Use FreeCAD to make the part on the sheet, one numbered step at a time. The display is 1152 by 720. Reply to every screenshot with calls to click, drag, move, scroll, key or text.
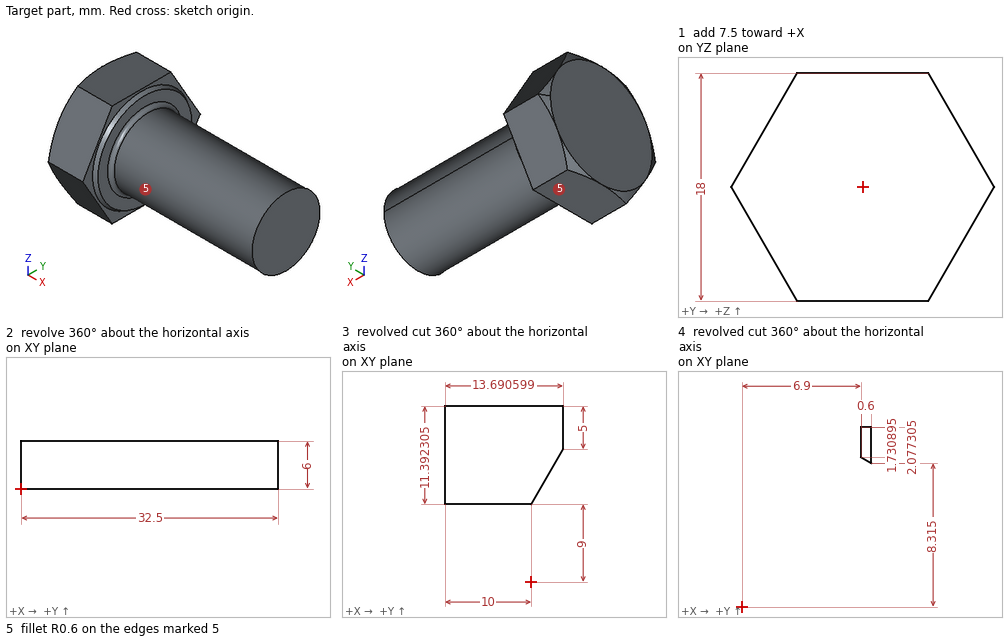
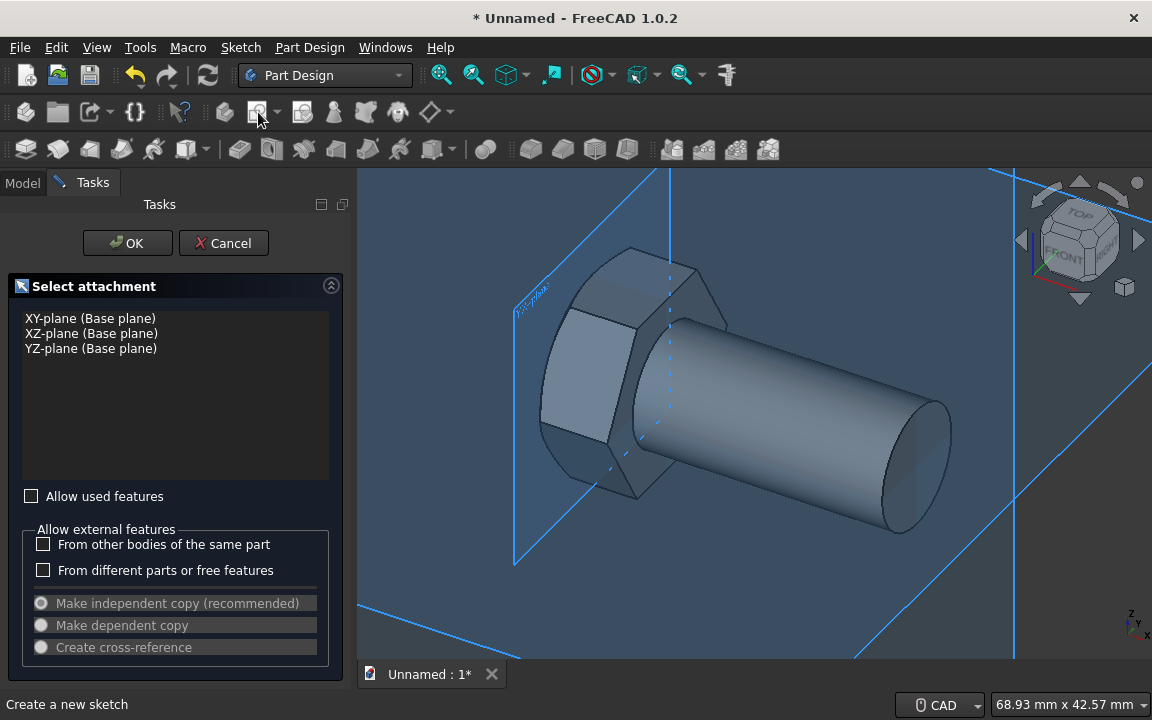
click(82, 318)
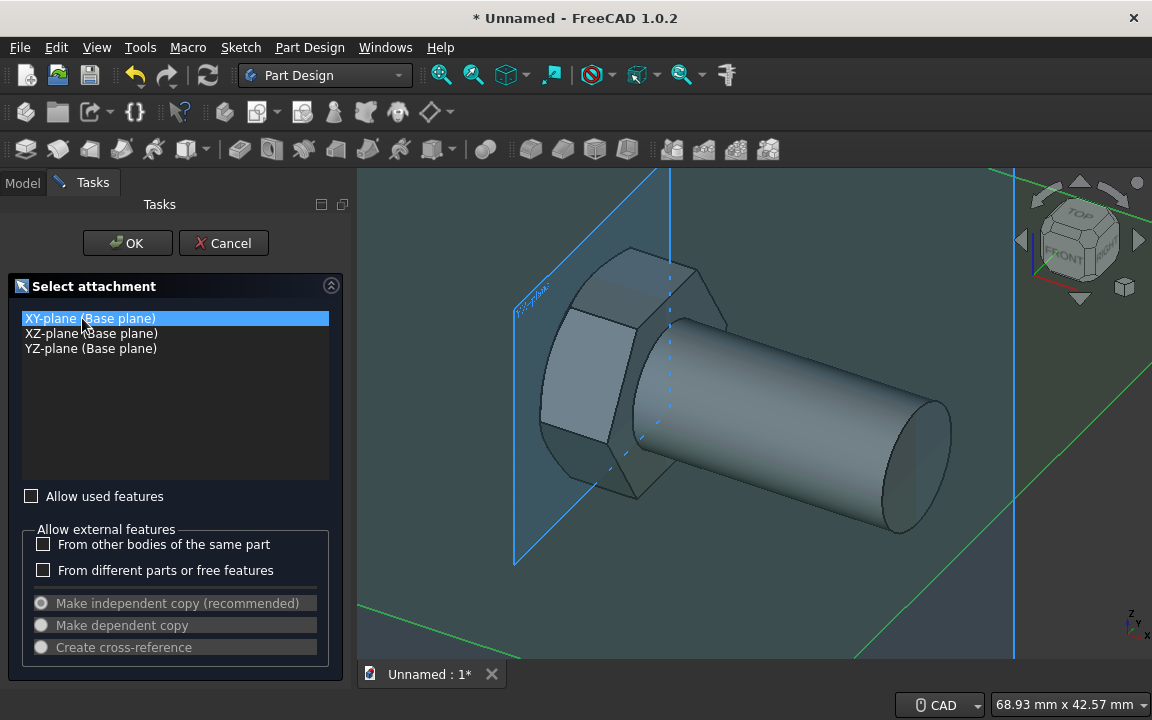
click(128, 243)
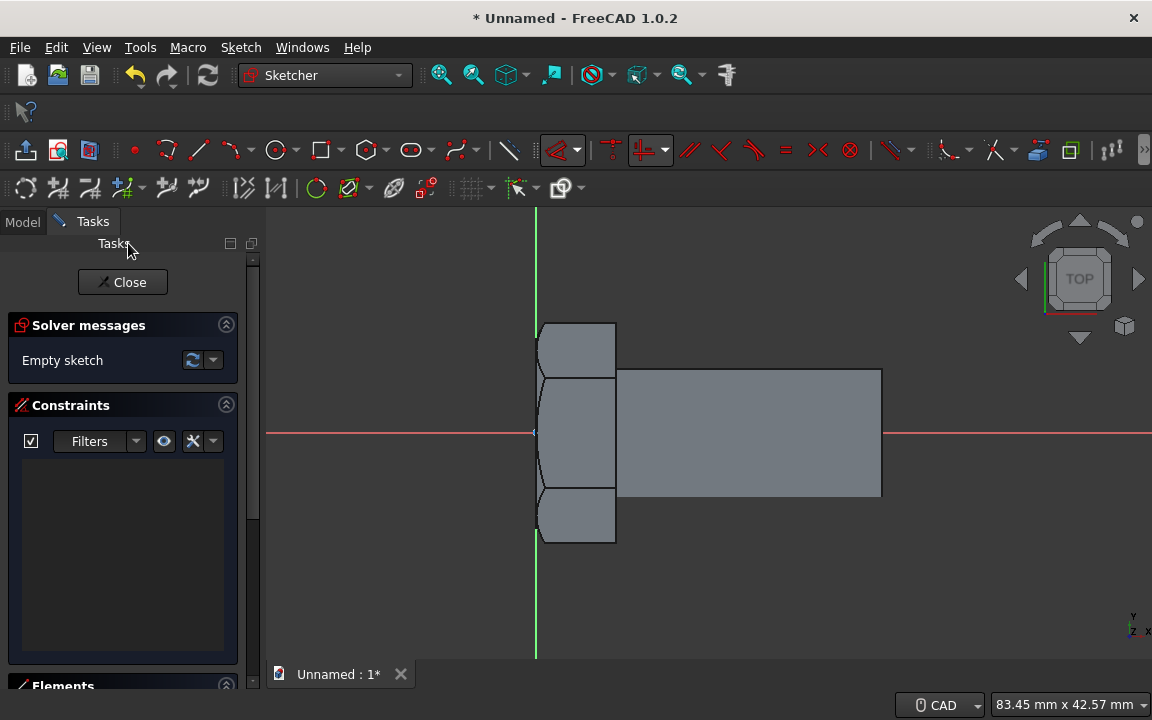
click(90, 150)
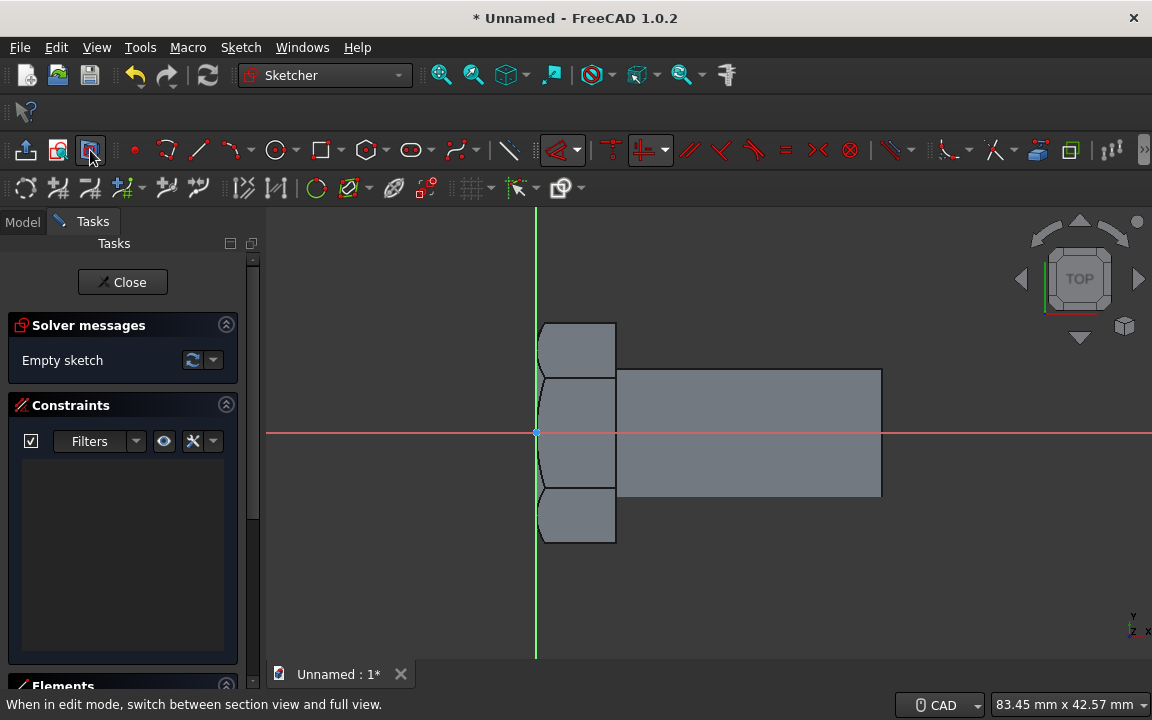
scroll(611, 326, up, 13)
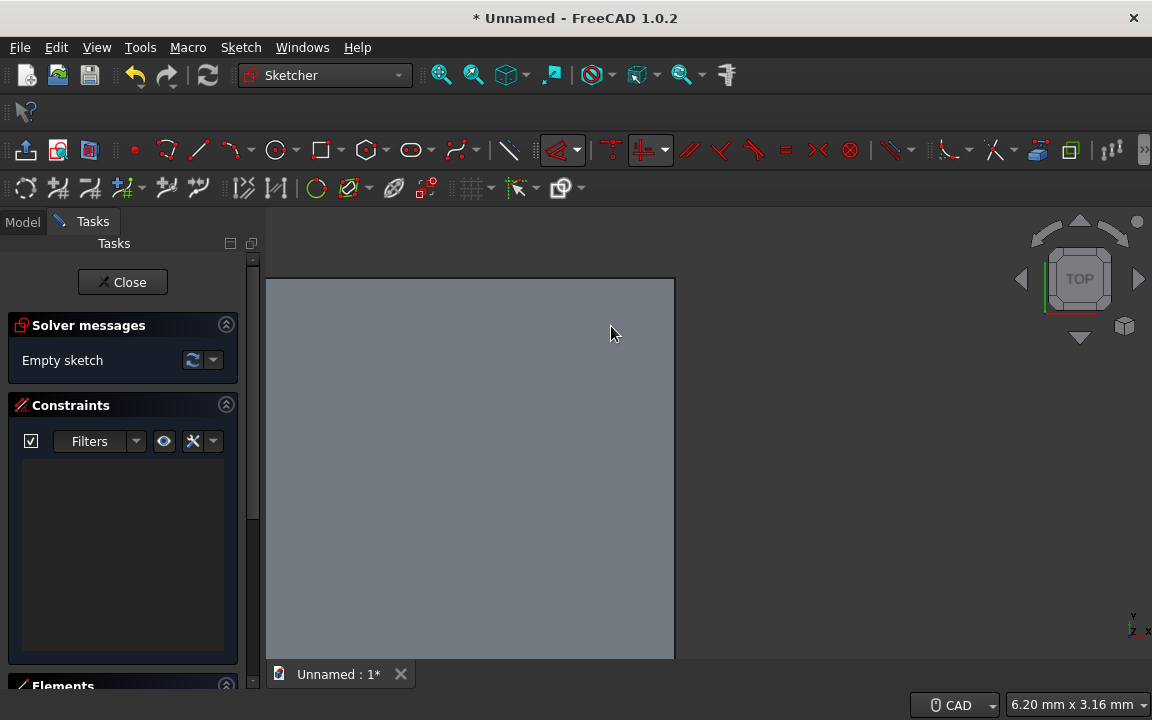
click(168, 150)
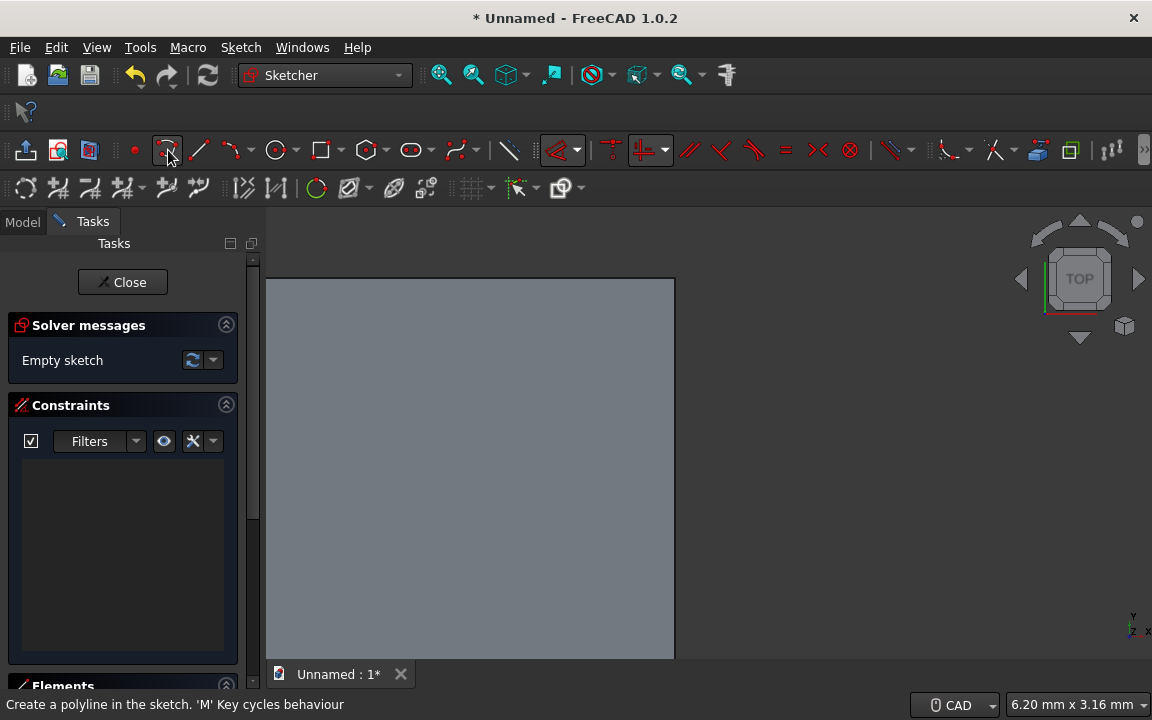
click(589, 525)
click(675, 575)
click(675, 278)
click(589, 278)
click(589, 526)
key(Escape)
key(Escape)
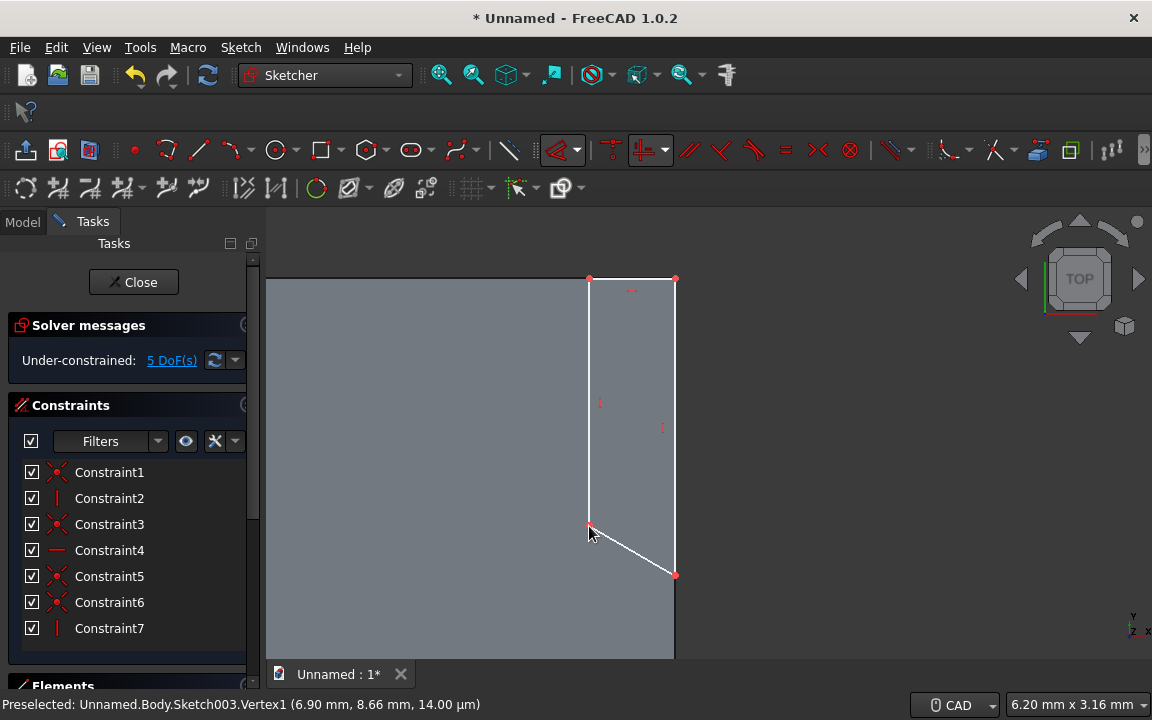
click(649, 279)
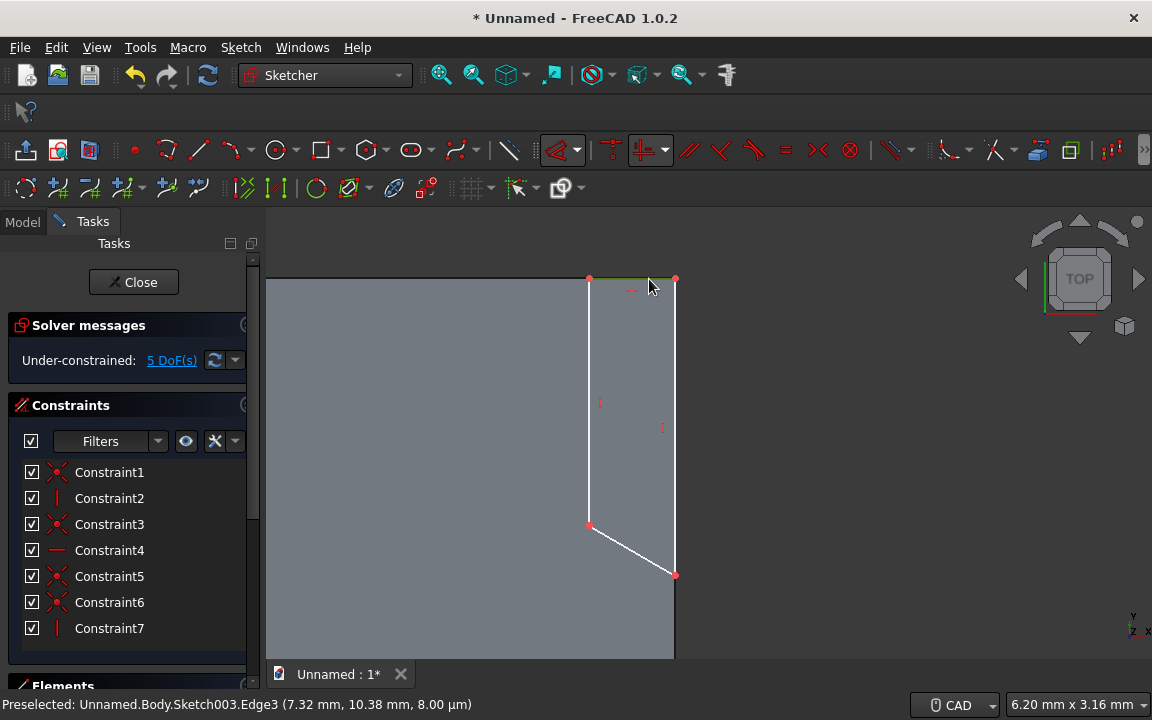
key(l)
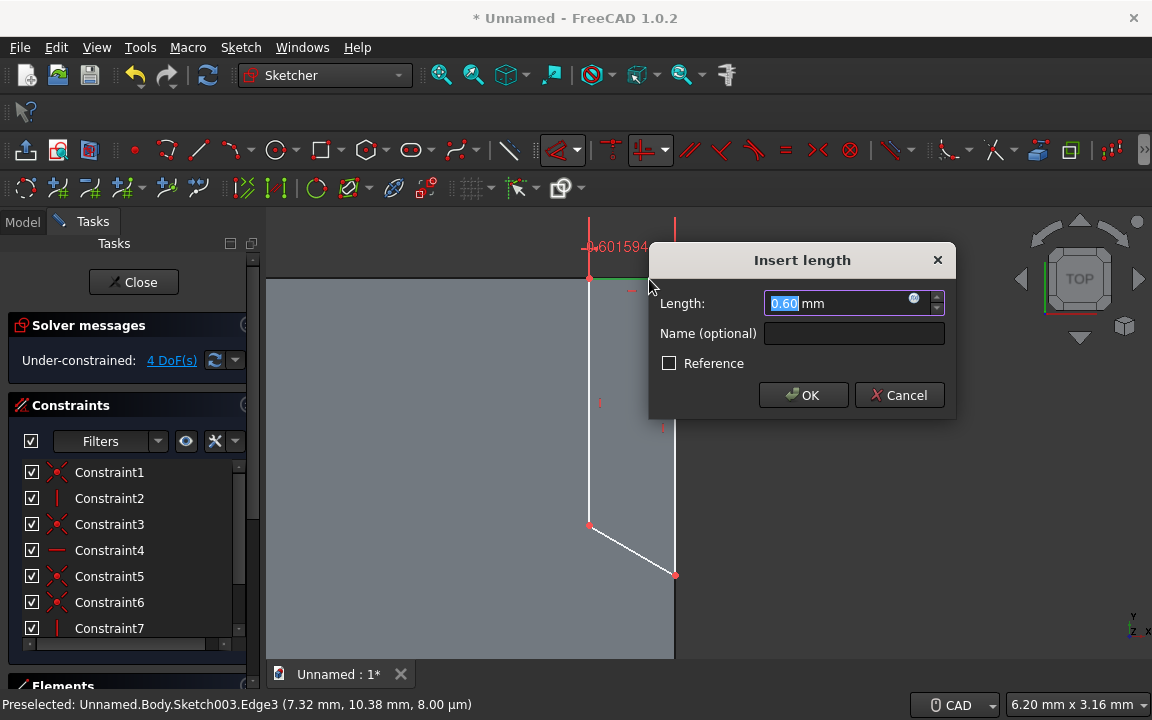
text(0.6)
key(Return)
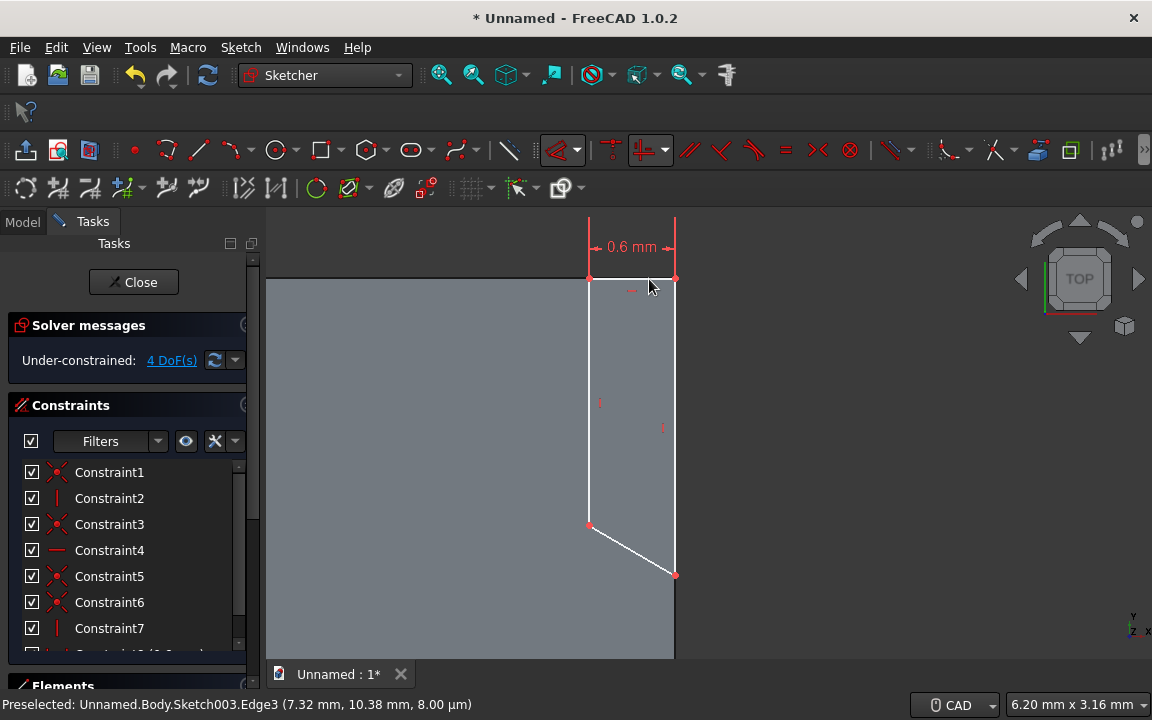
click(589, 526)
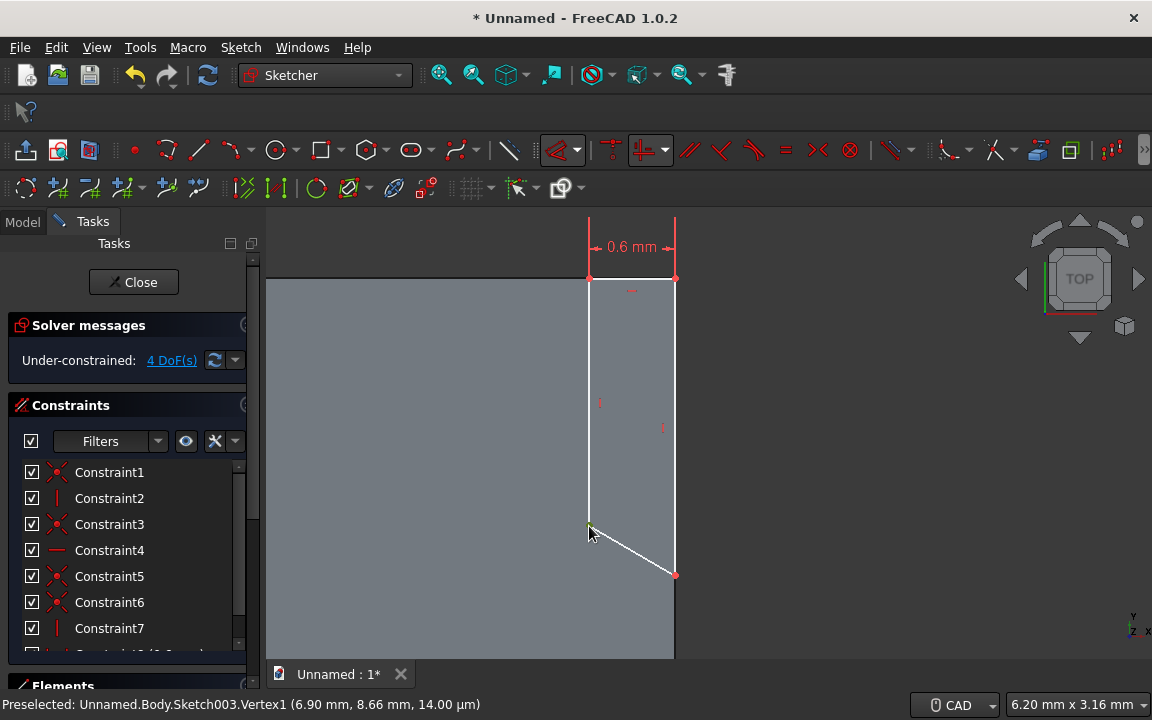
key(l)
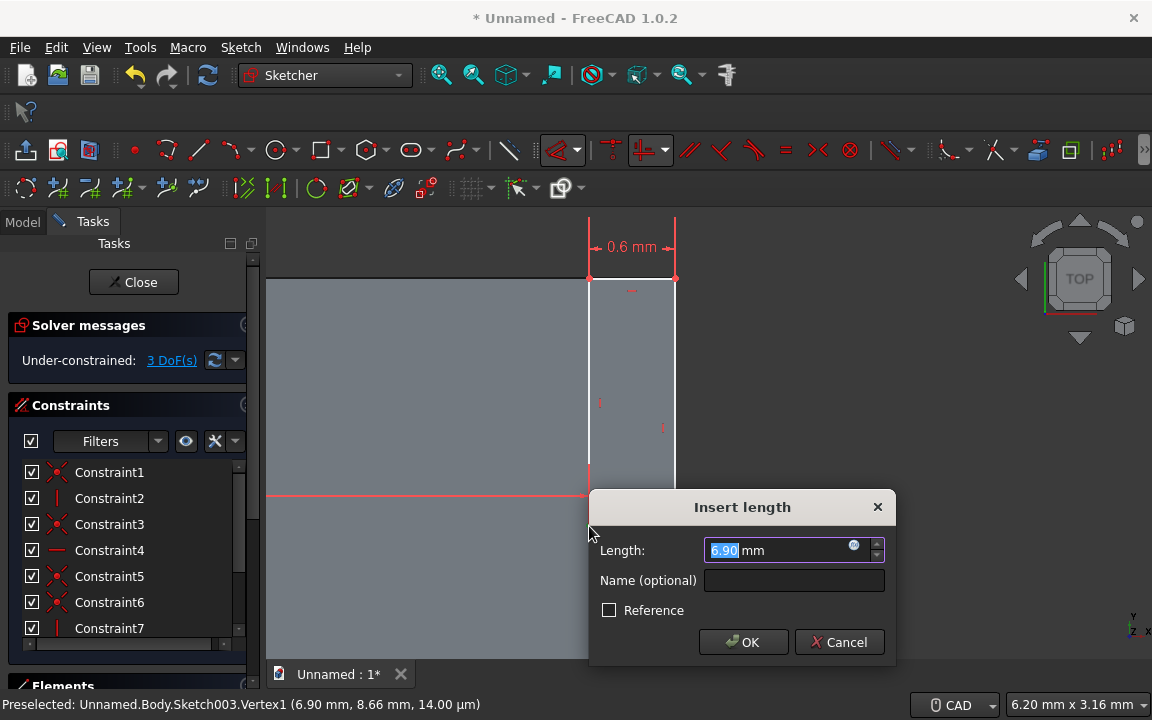
text(6.9)
key(Return)